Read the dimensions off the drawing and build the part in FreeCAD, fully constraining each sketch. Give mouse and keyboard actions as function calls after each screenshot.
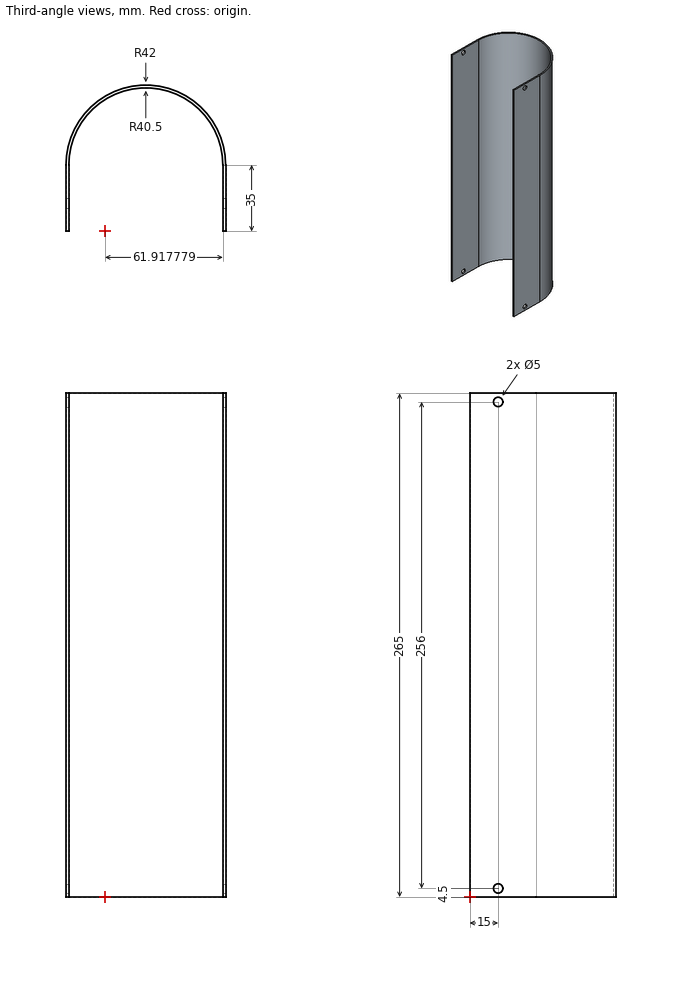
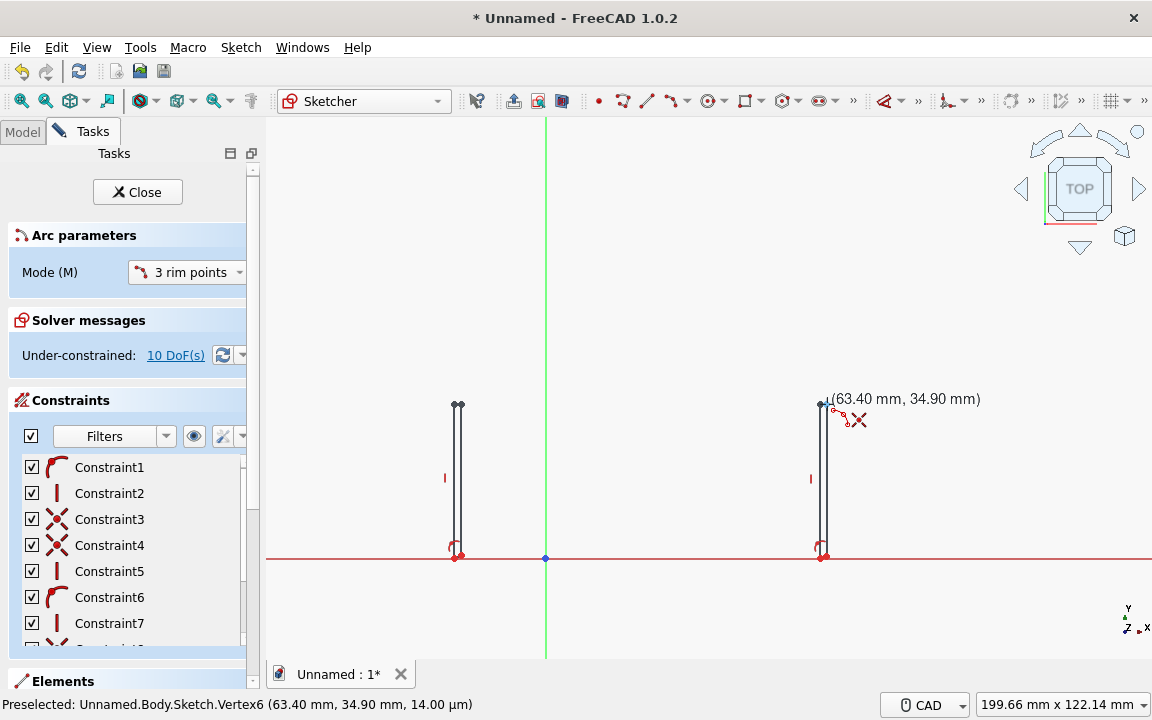
scroll(454, 404, up, 5)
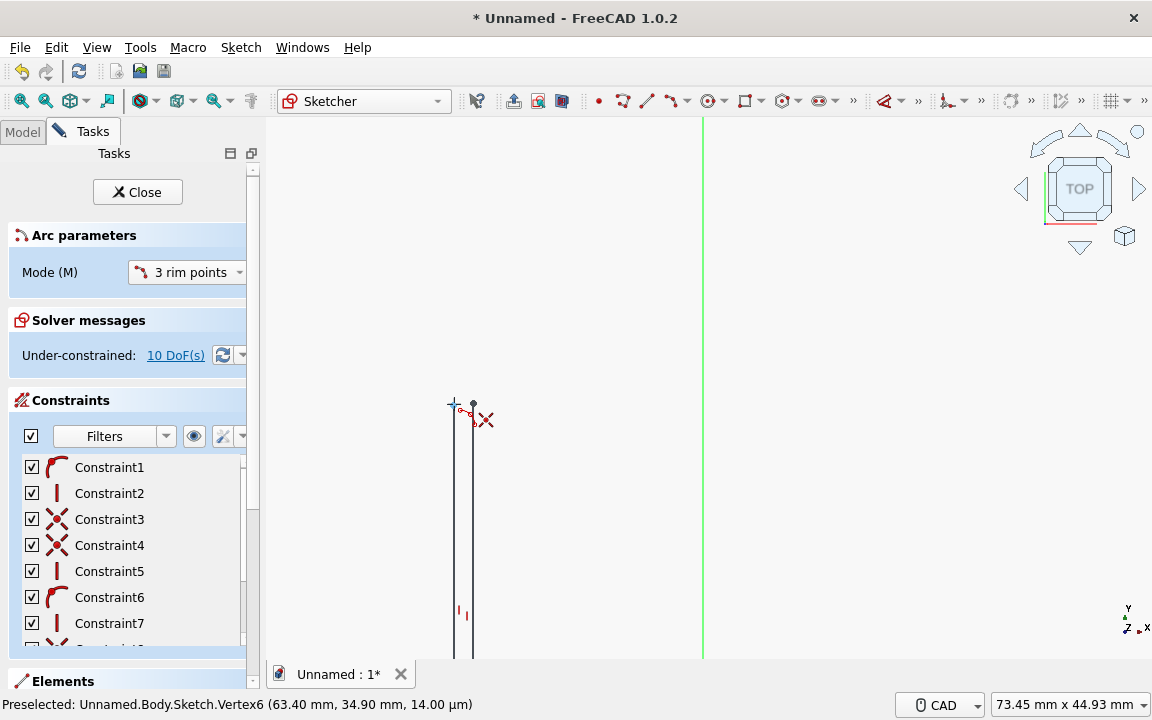
click(454, 406)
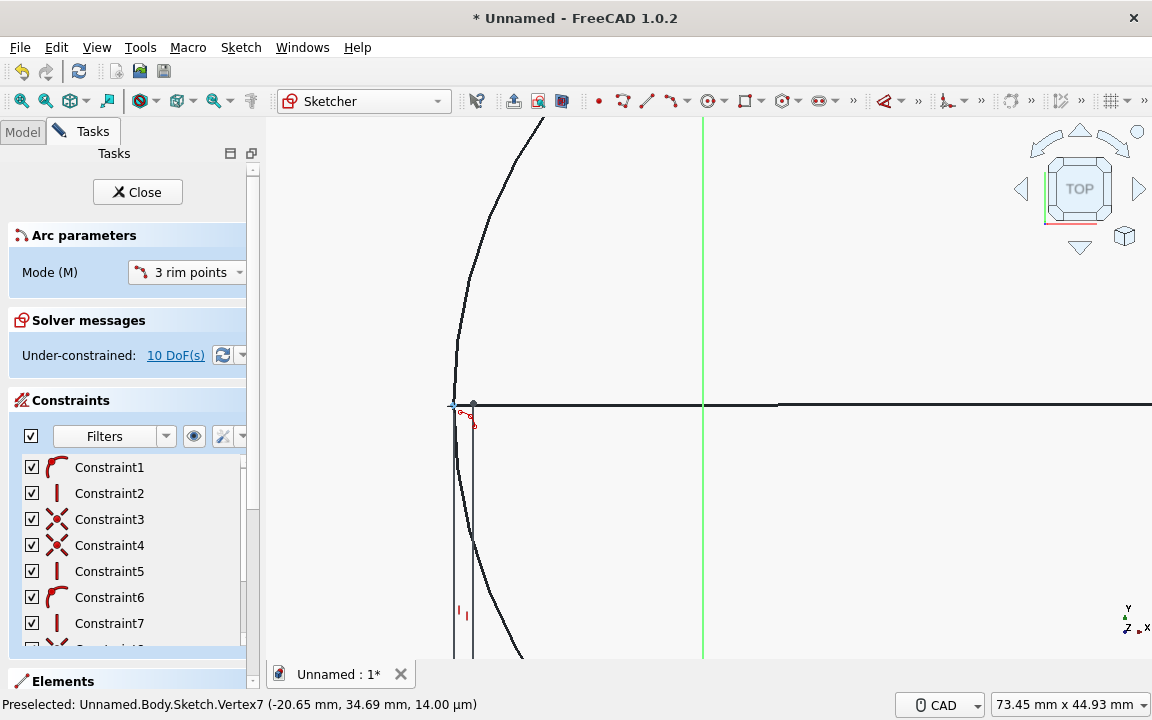
scroll(454, 404, down, 5)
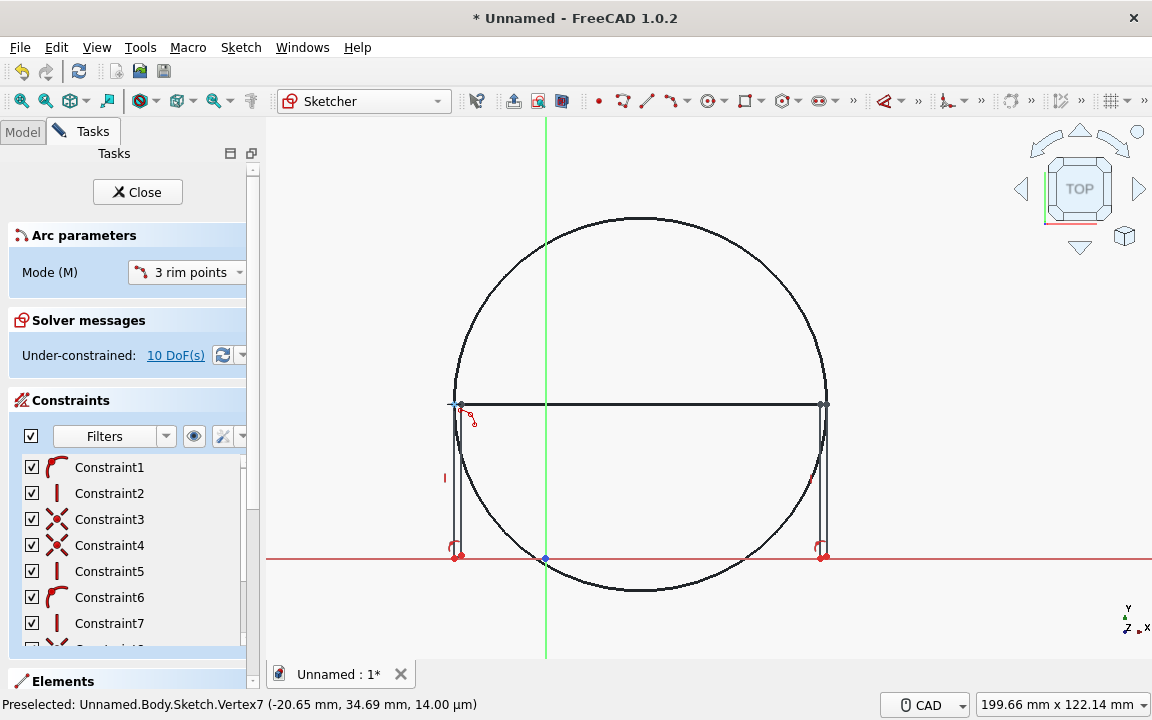
click(641, 217)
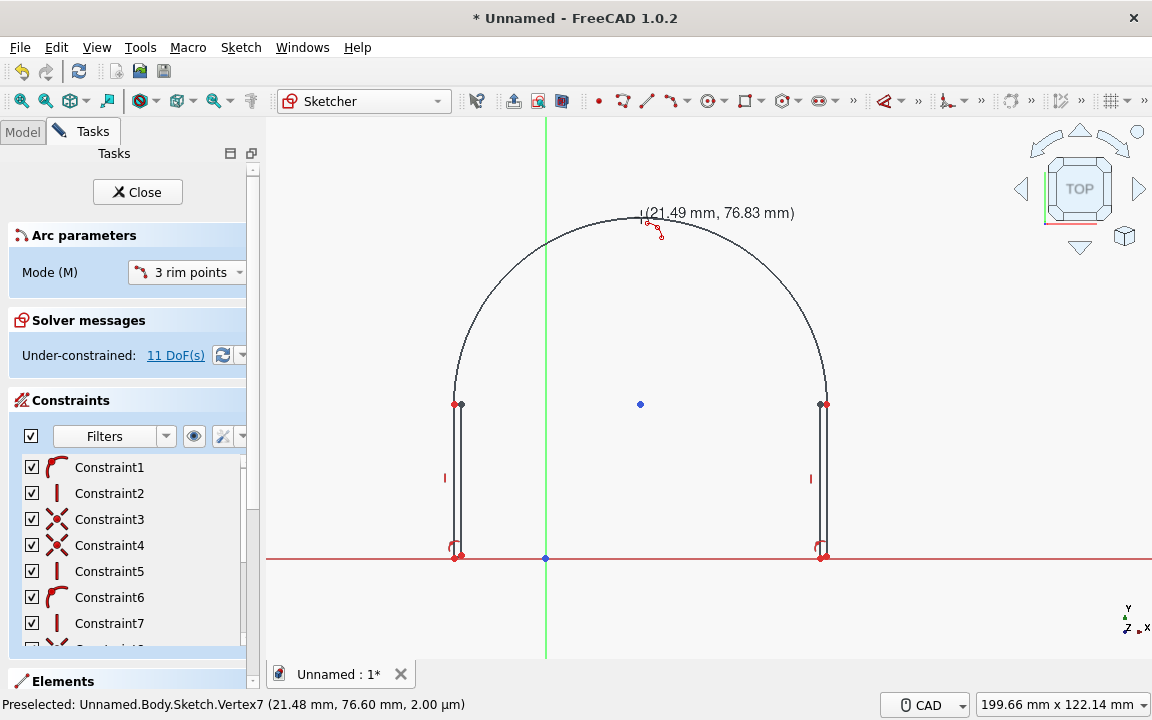
scroll(461, 404, up, 5)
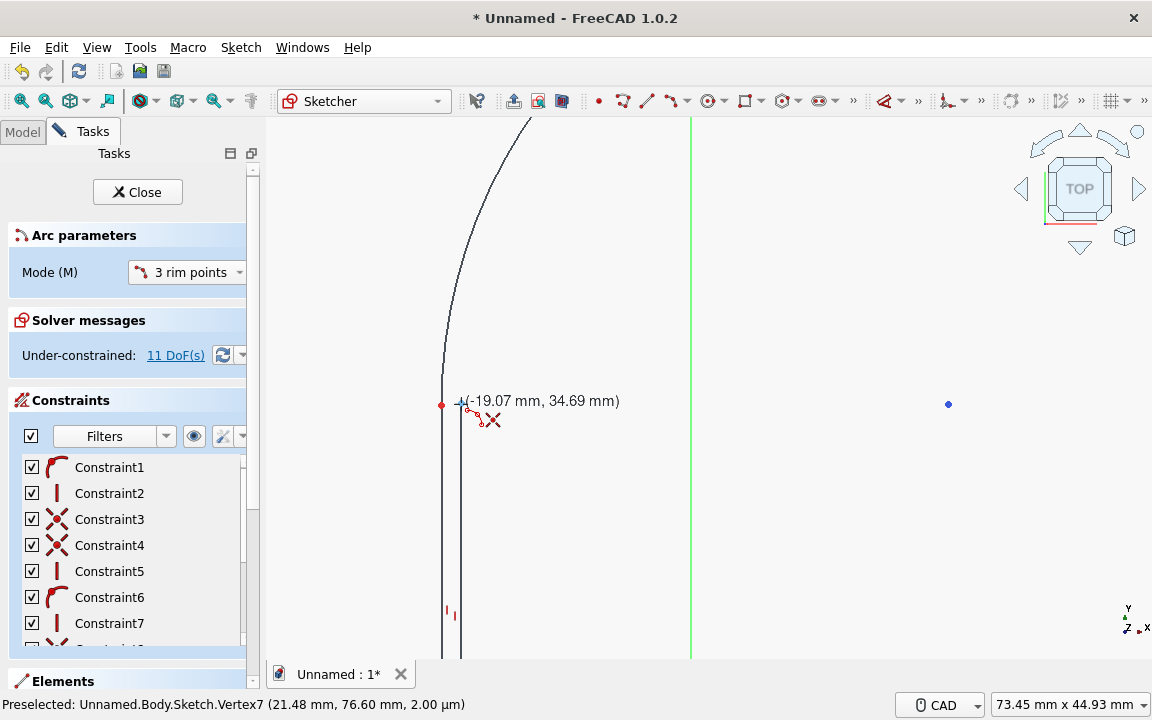
click(461, 403)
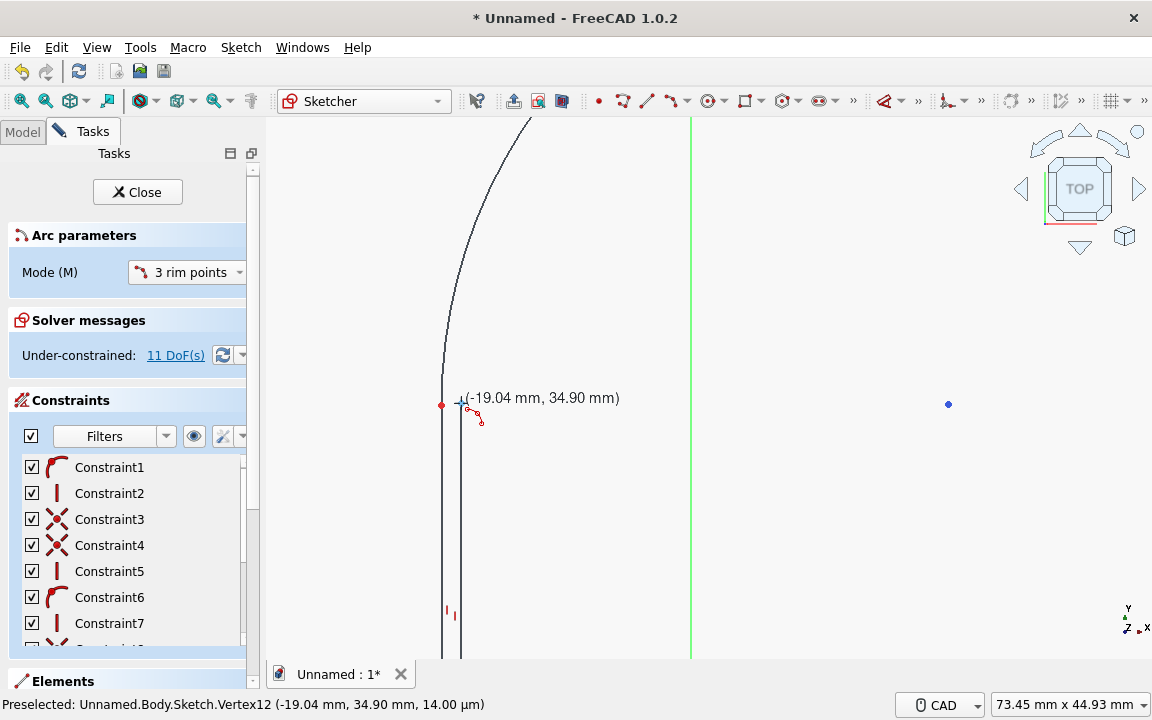
scroll(461, 404, down, 5)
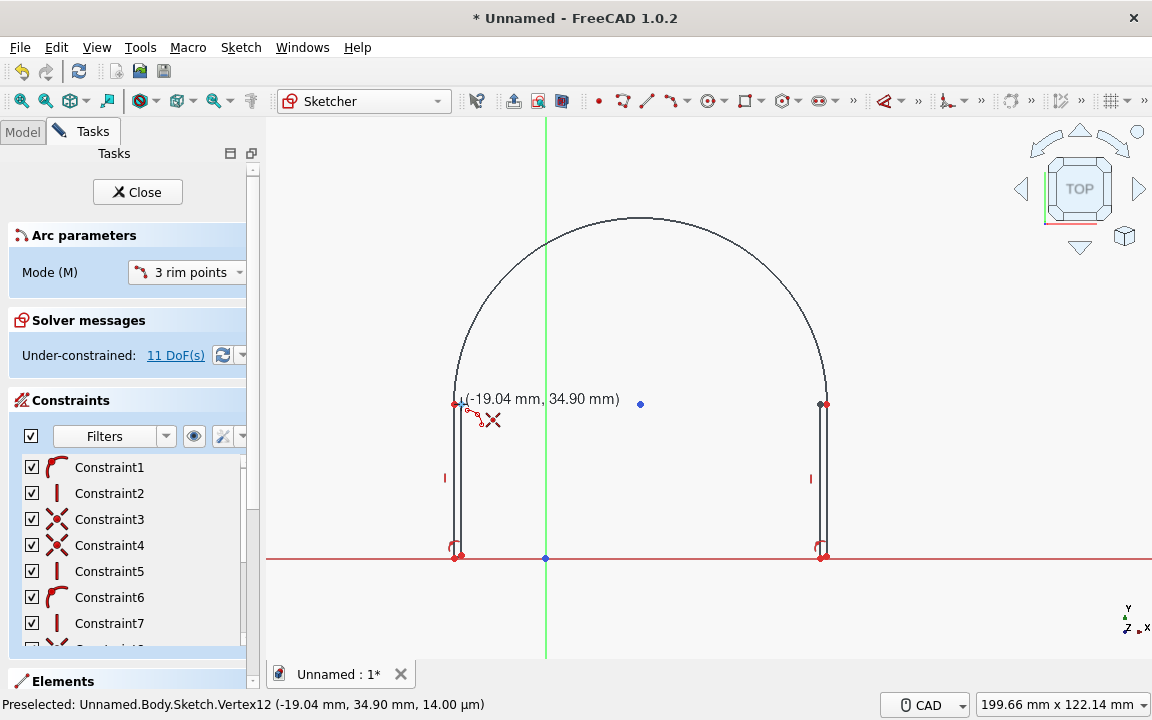
scroll(820, 404, up, 5)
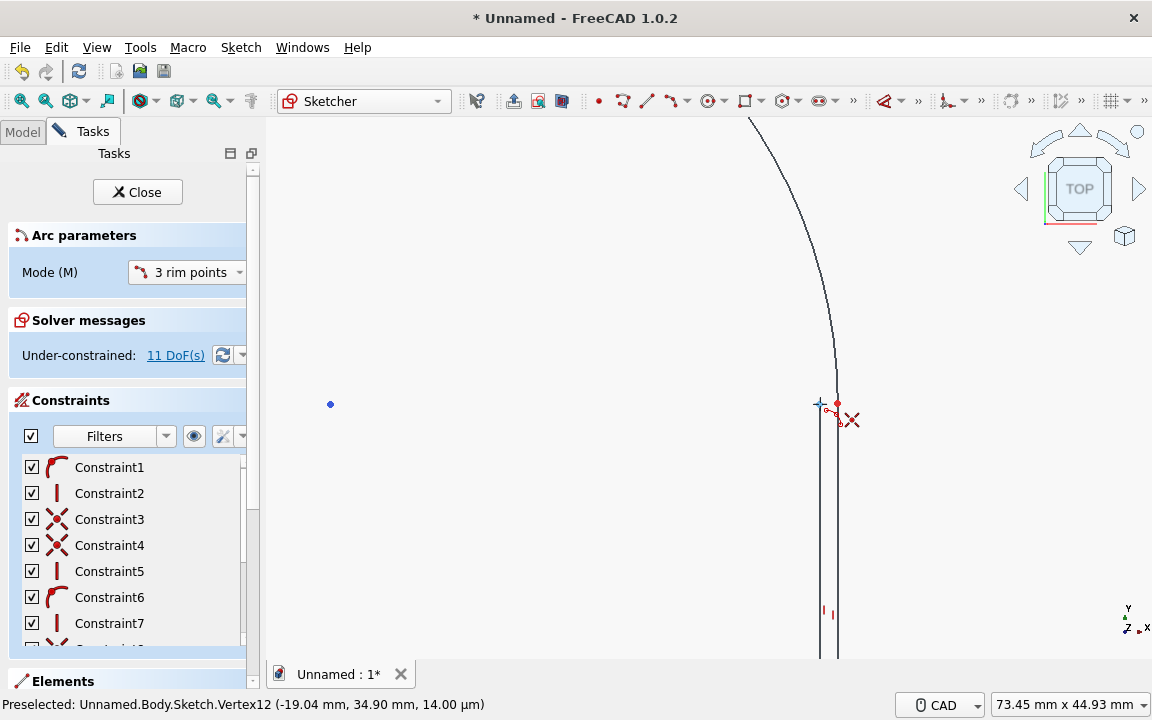
click(820, 405)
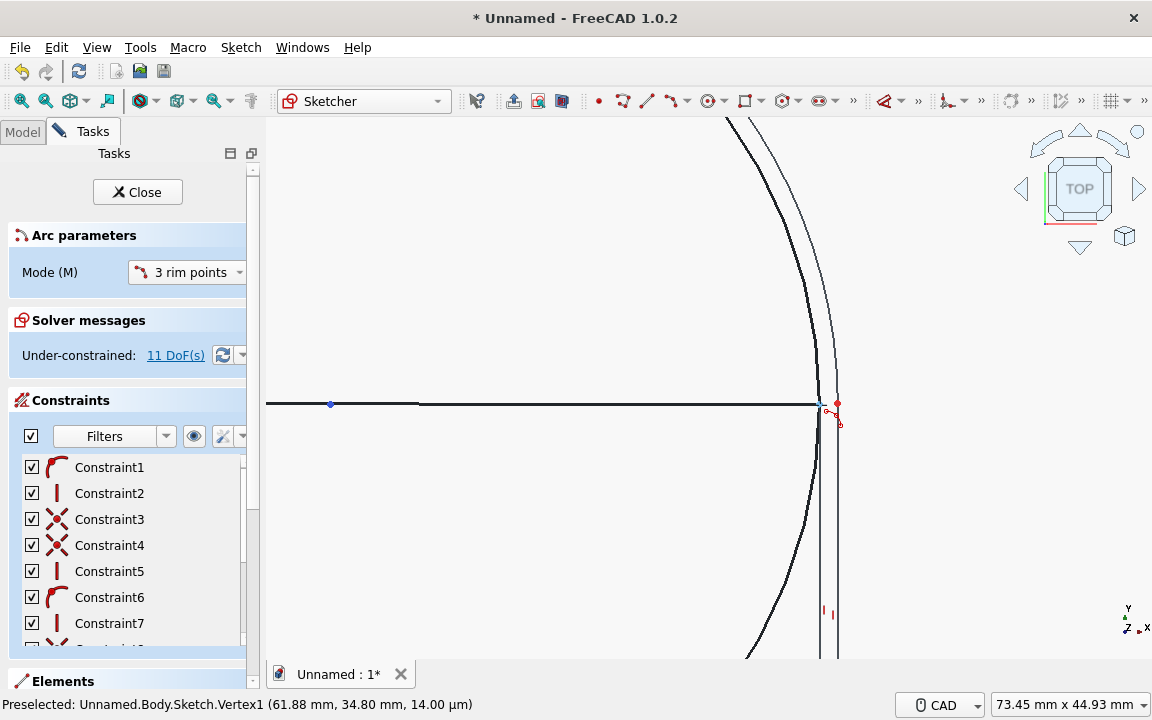
scroll(820, 404, down, 5)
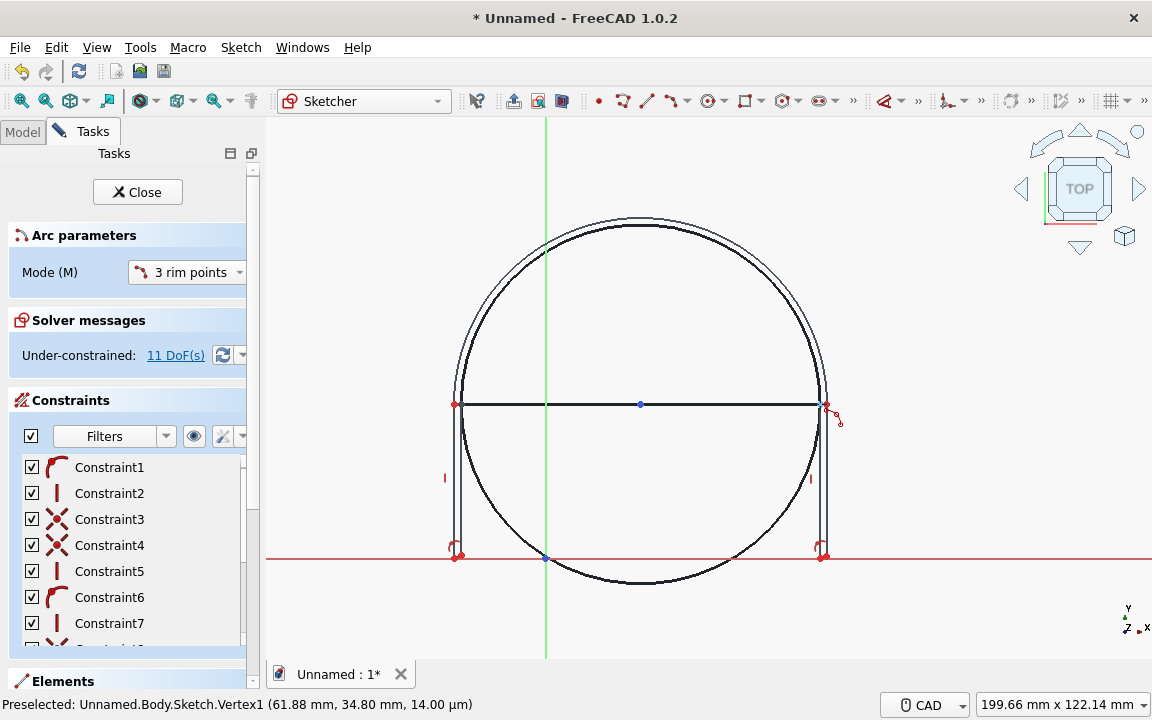
scroll(696, 233, up, 5)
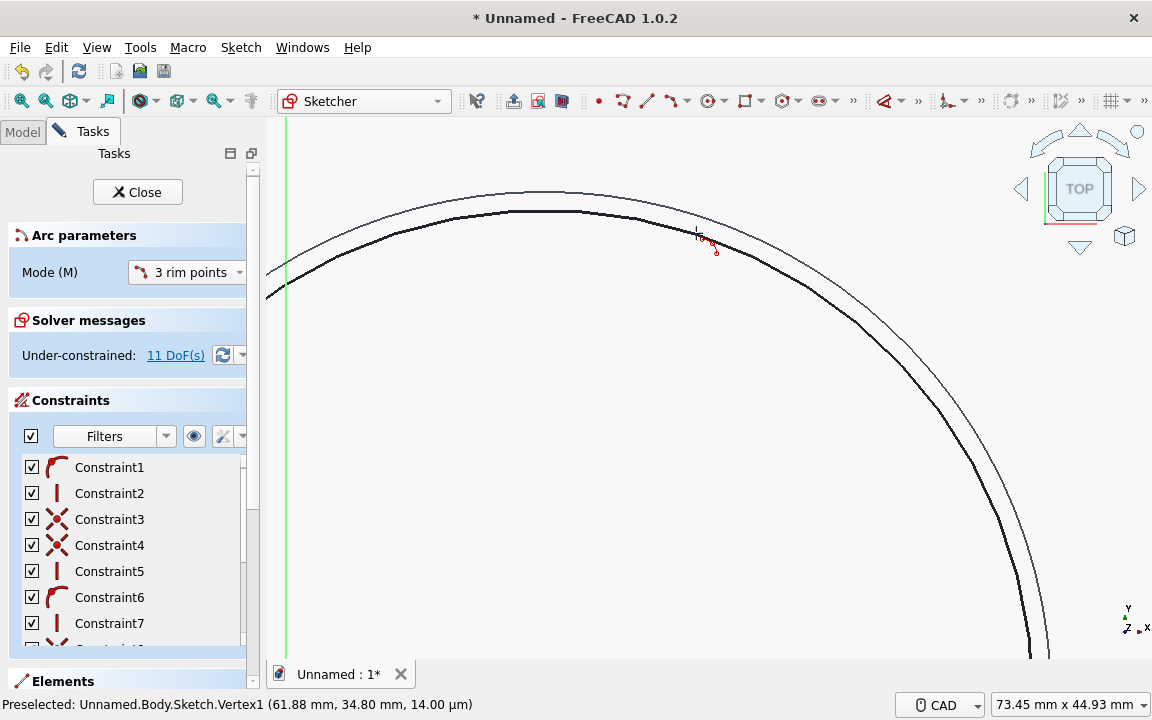
click(696, 232)
key(Escape)